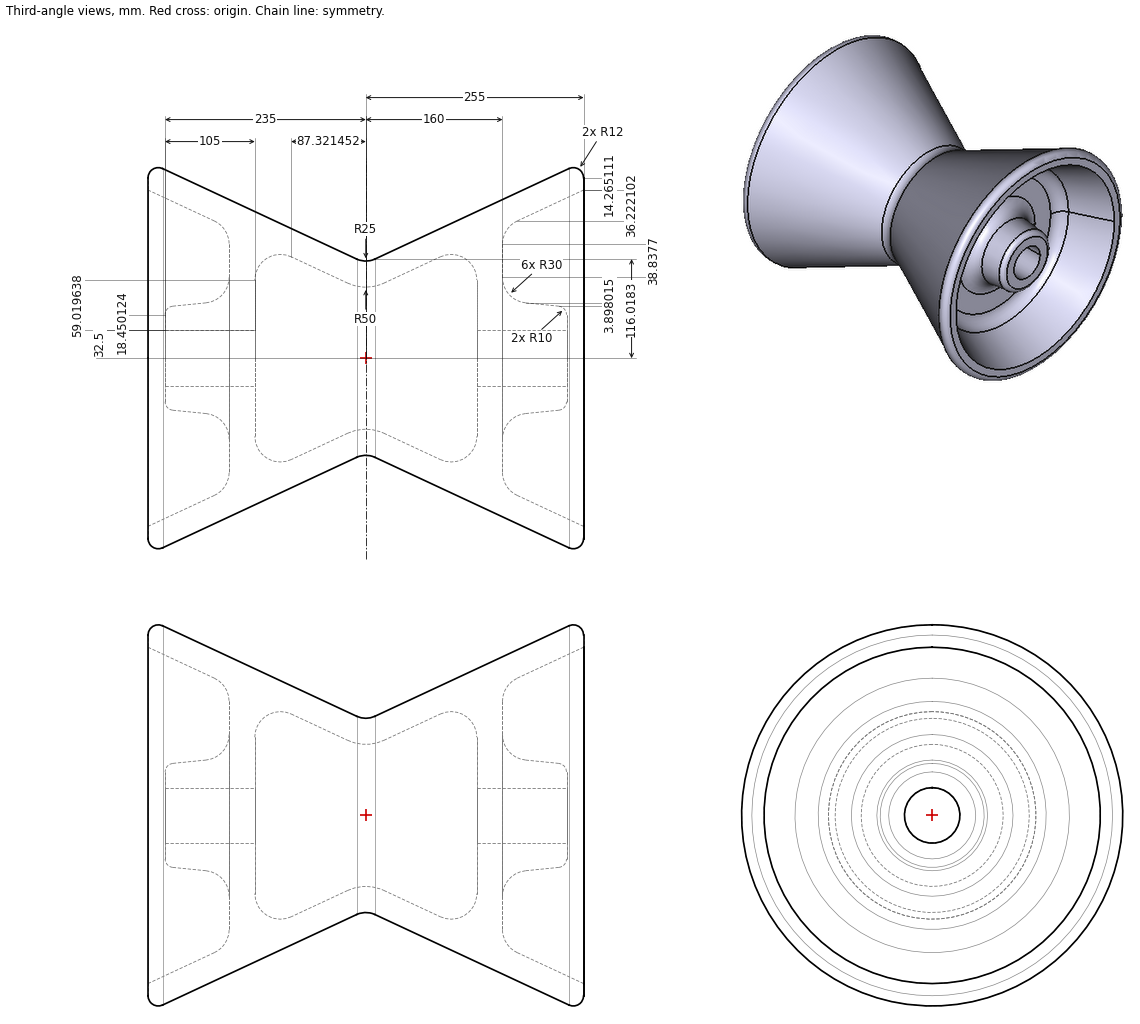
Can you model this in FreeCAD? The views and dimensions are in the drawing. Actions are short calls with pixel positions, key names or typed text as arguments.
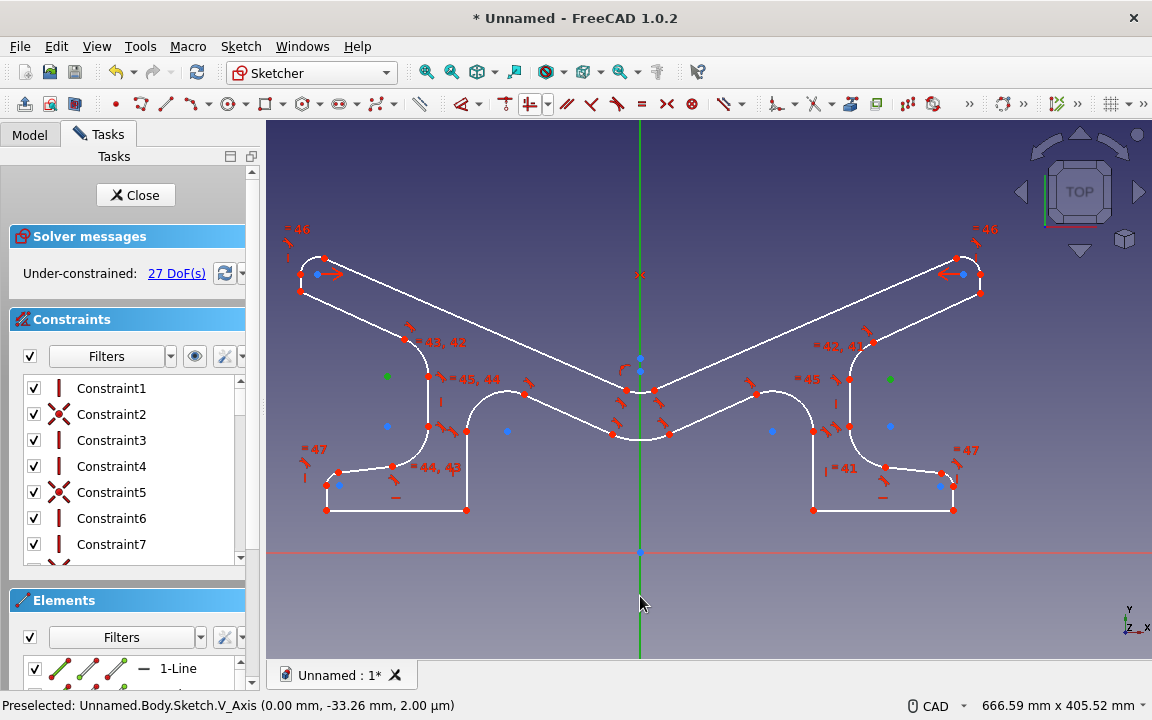
key(s)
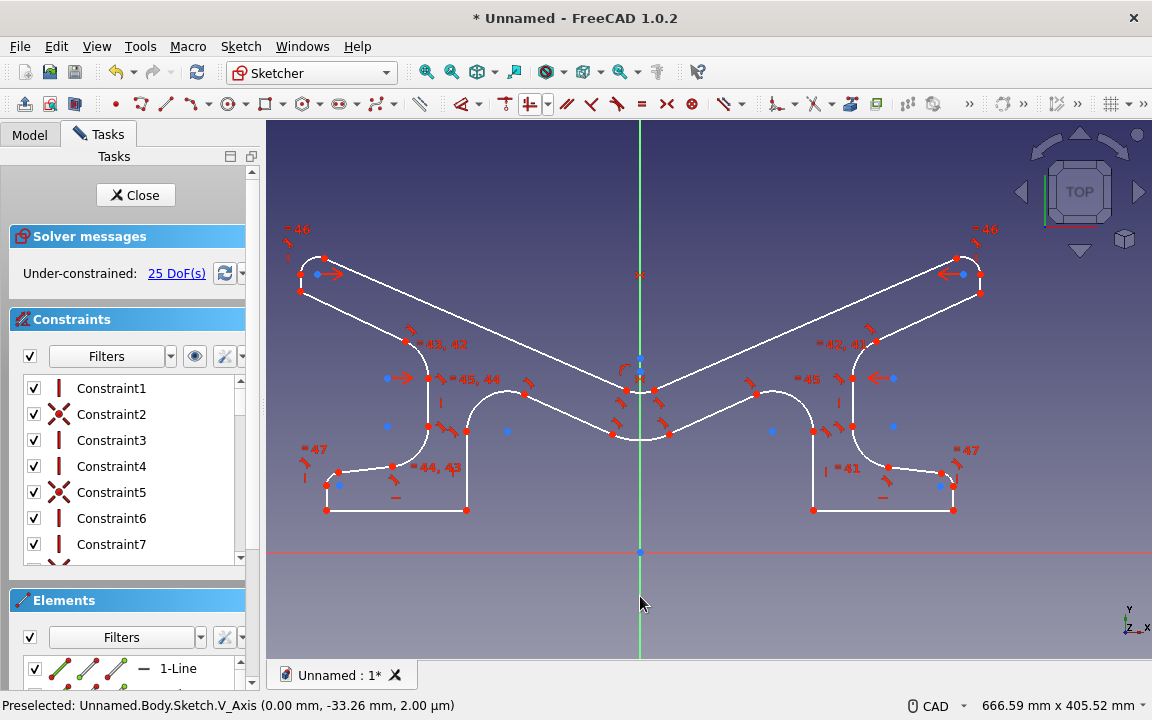
click(507, 432)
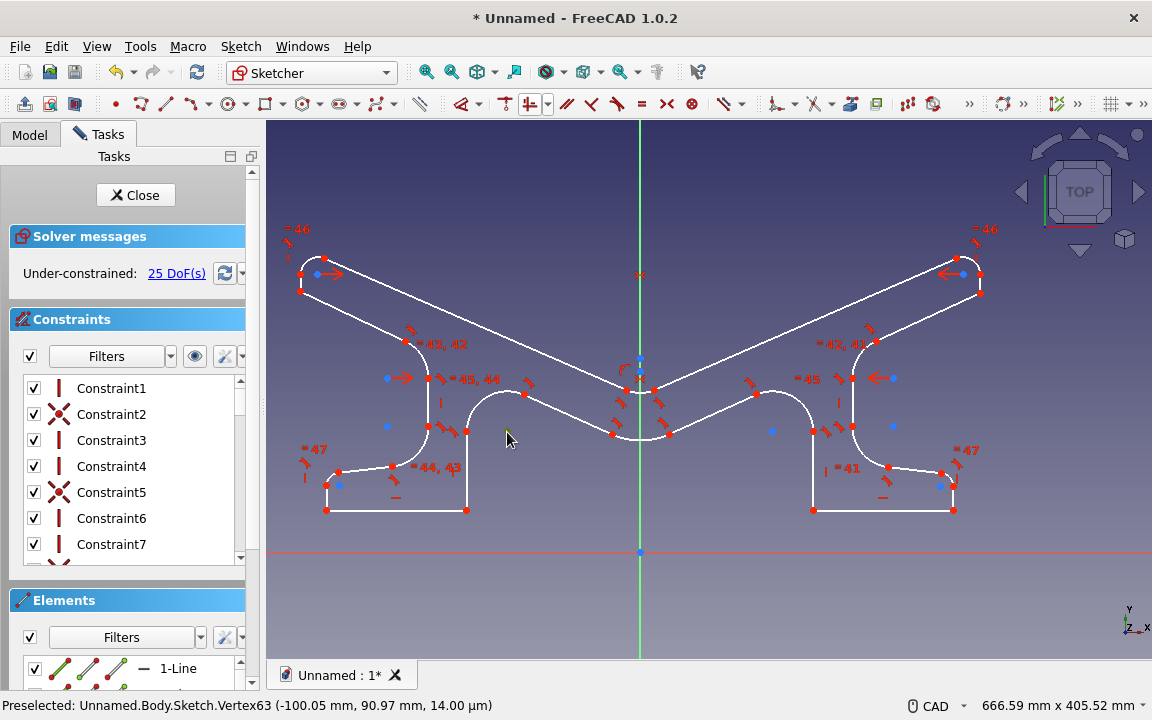
click(773, 432)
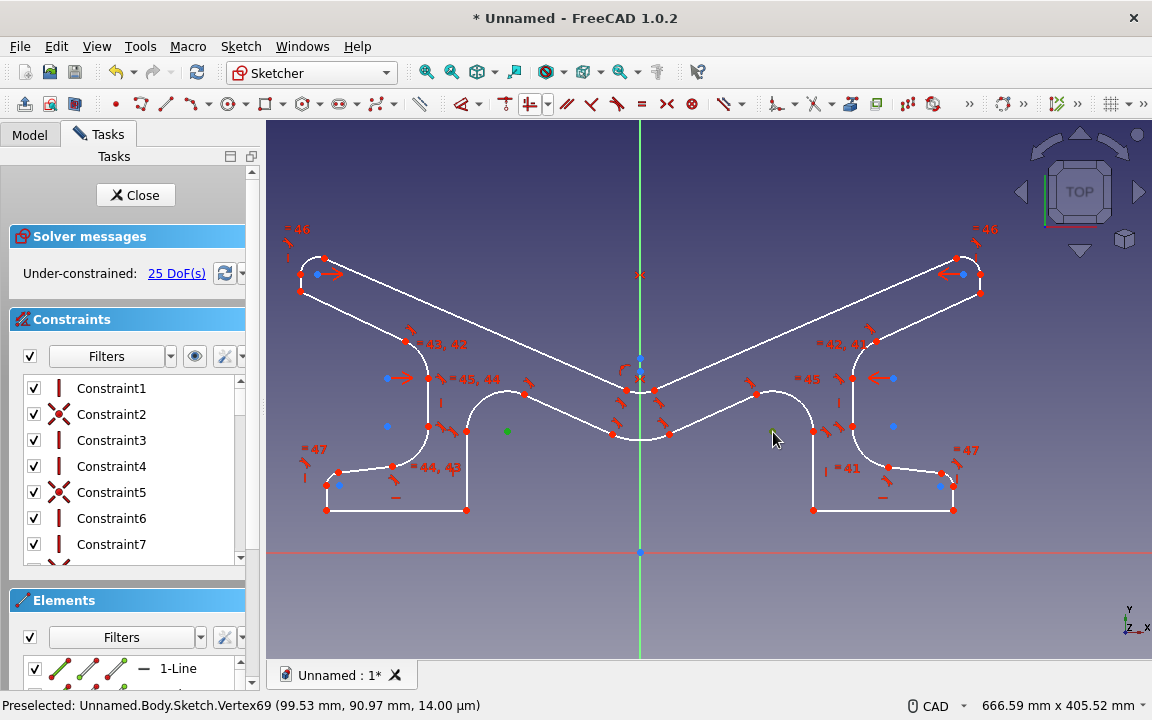
click(640, 596)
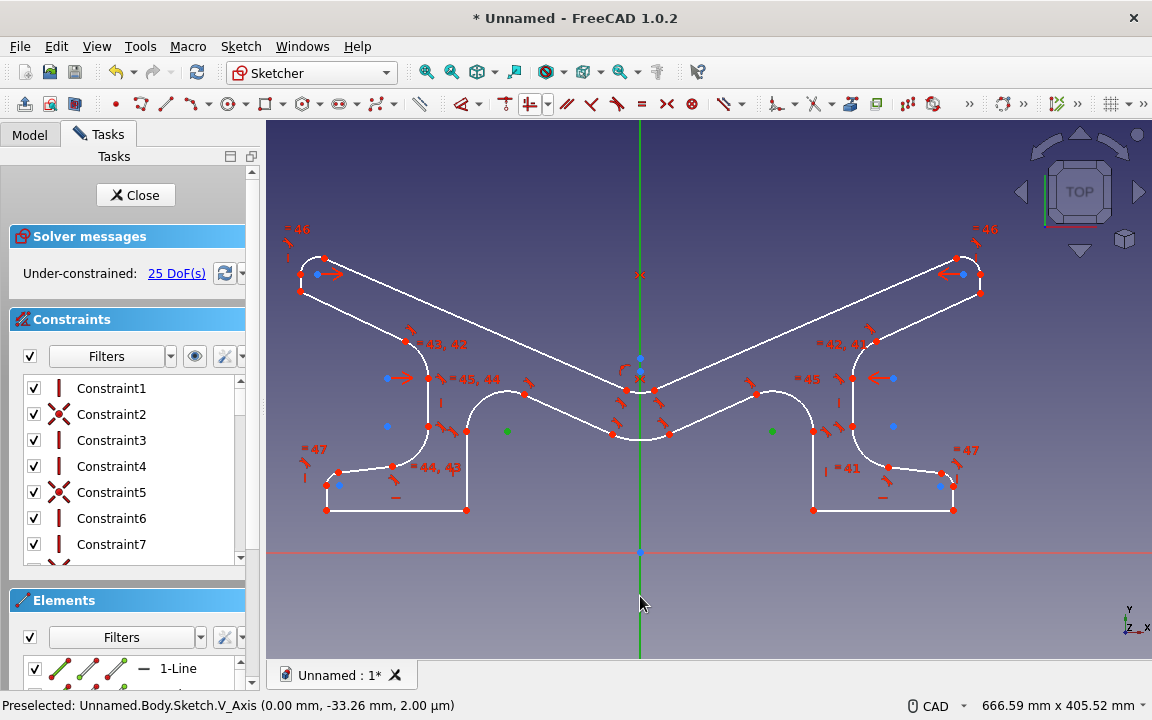
click(667, 104)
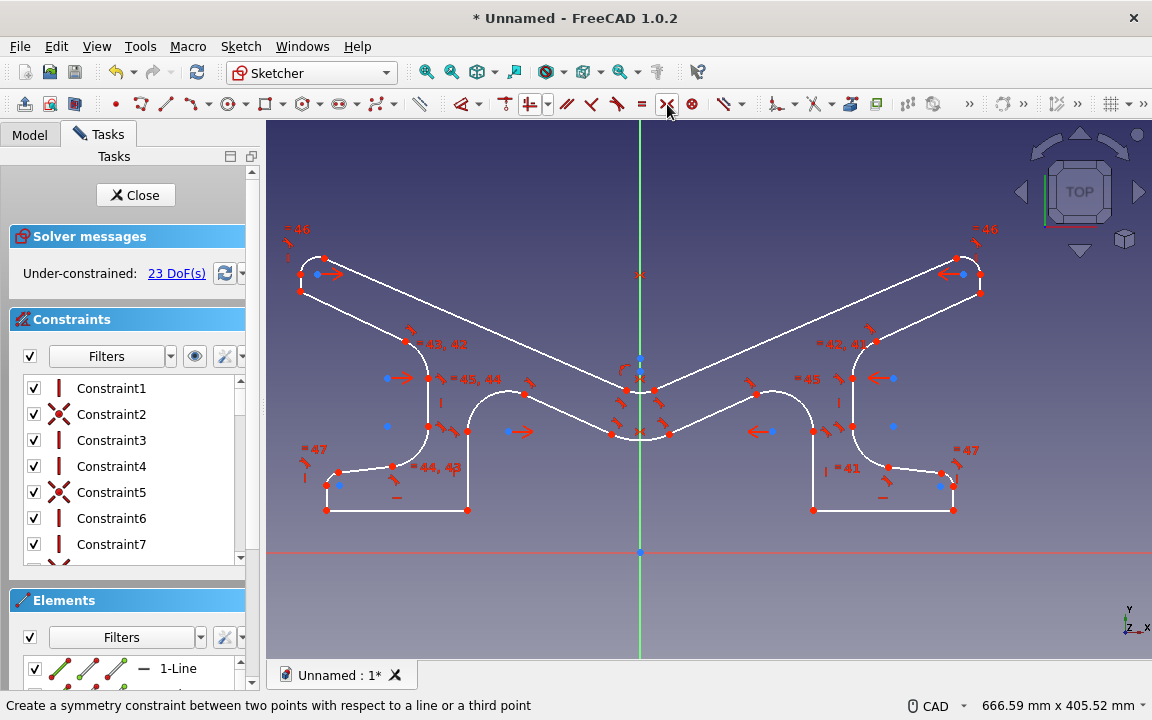
click(340, 486)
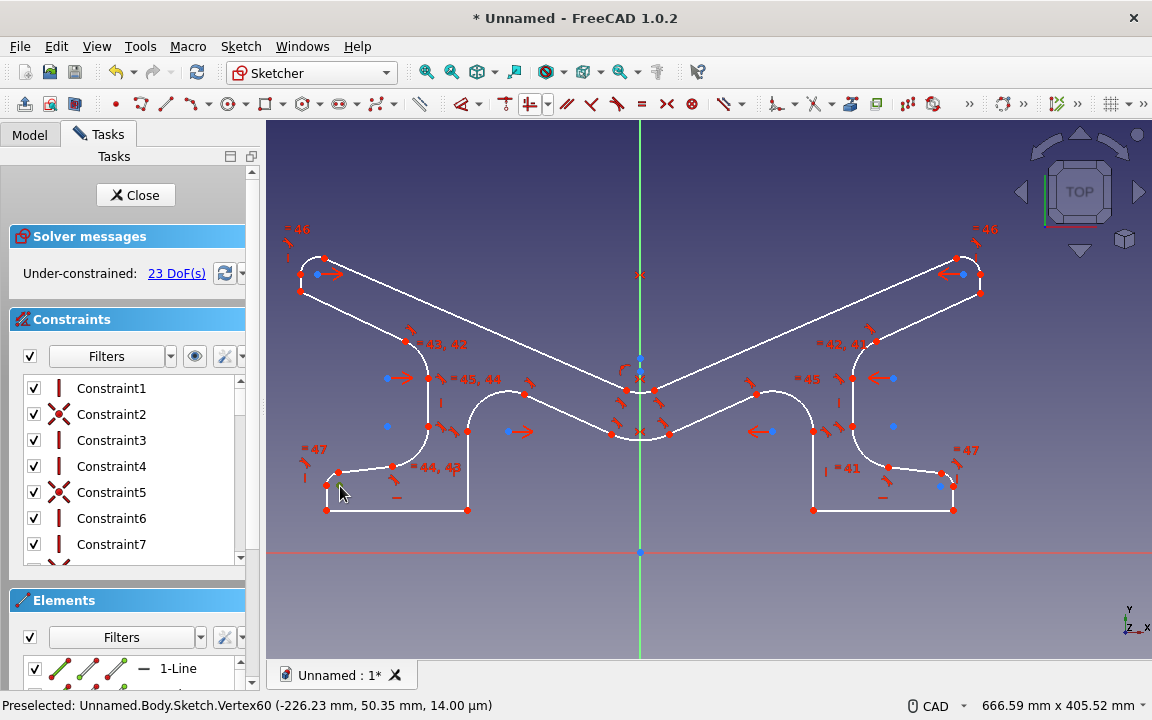
click(940, 486)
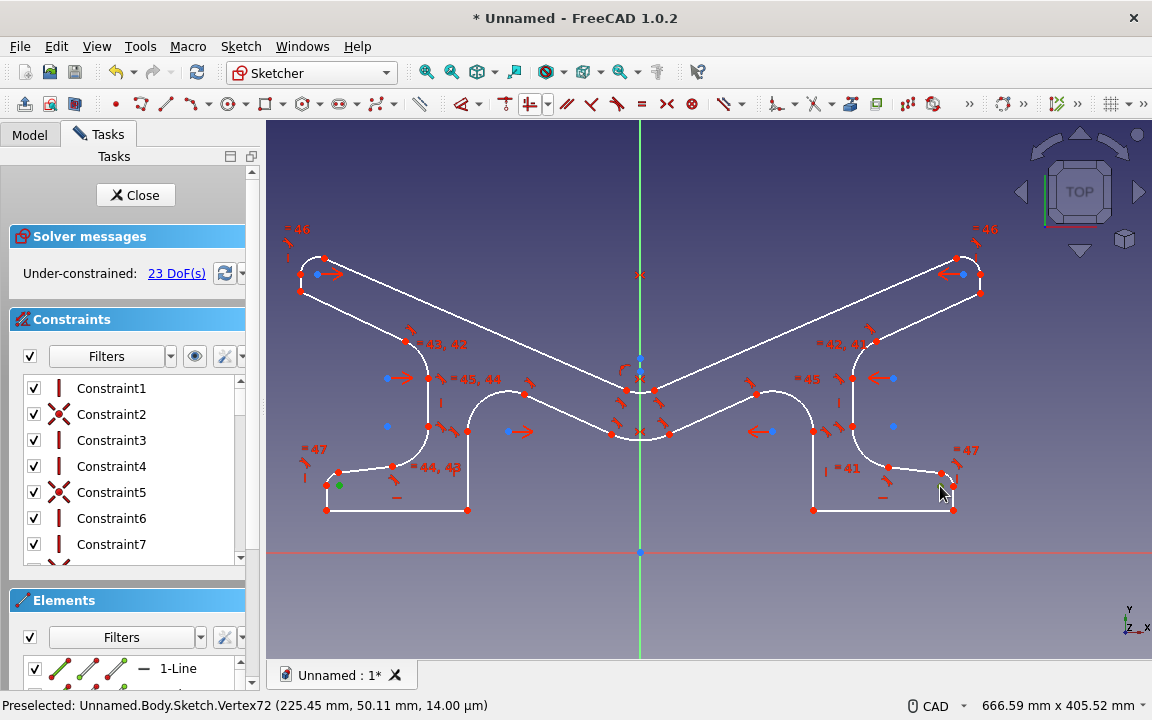
click(640, 596)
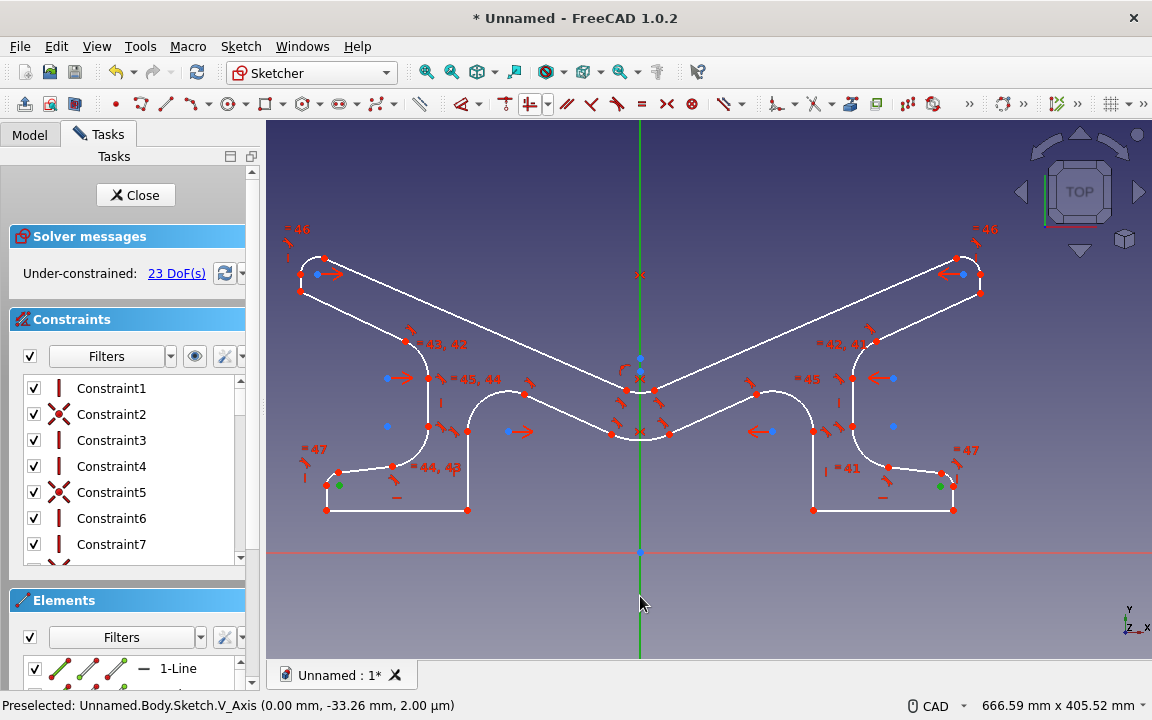
click(667, 104)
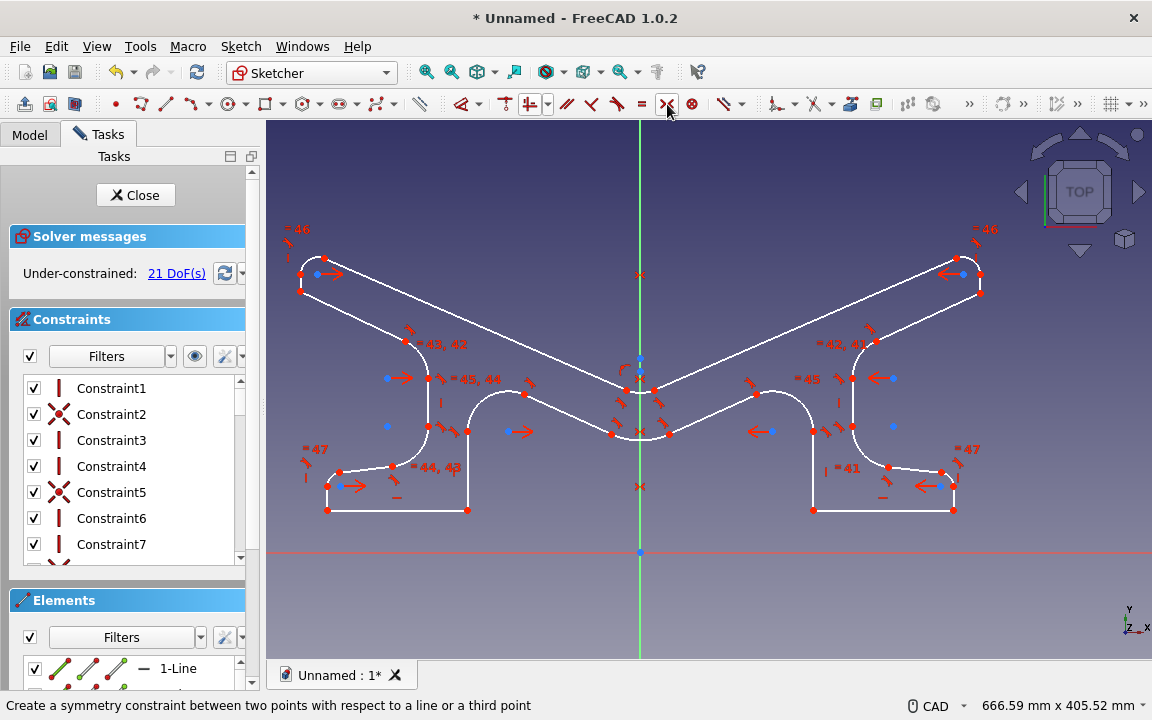
click(460, 104)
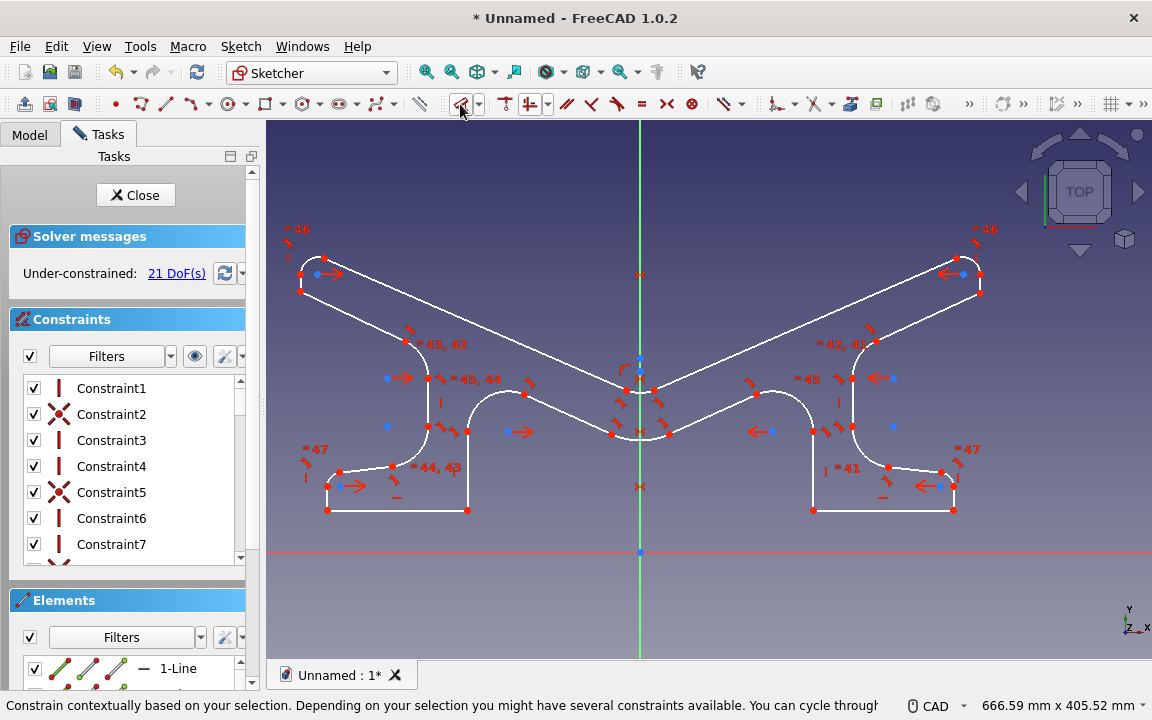
click(856, 444)
click(827, 457)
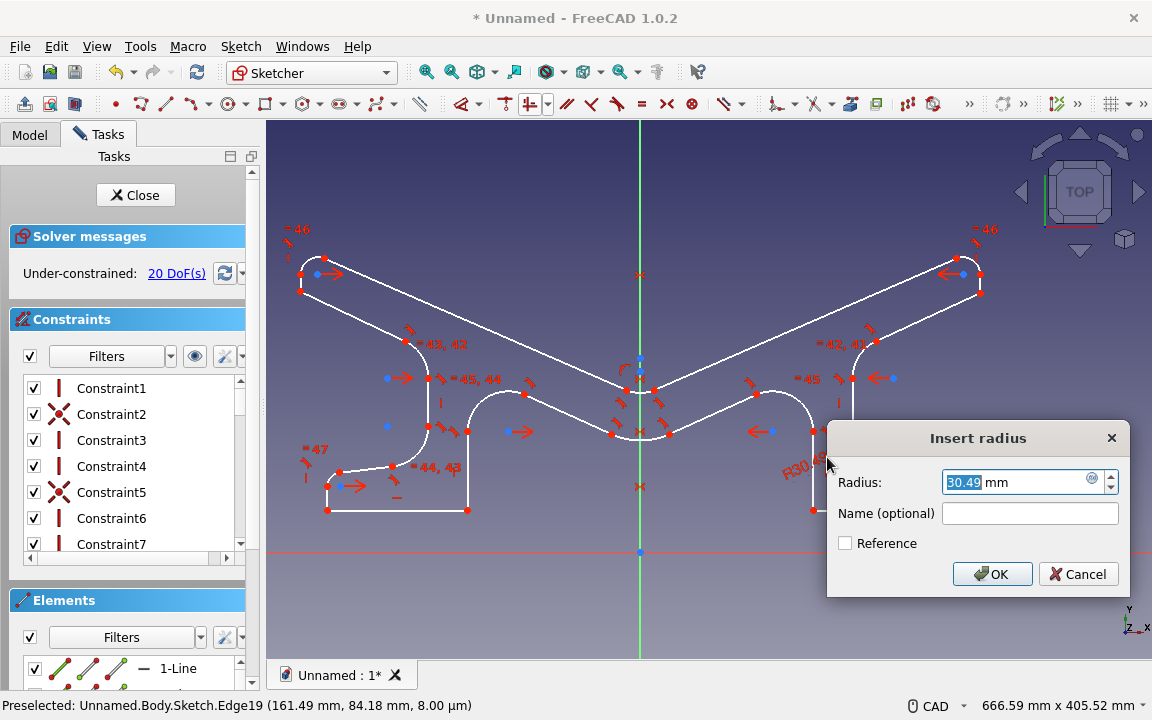
text(30)
key(Return)